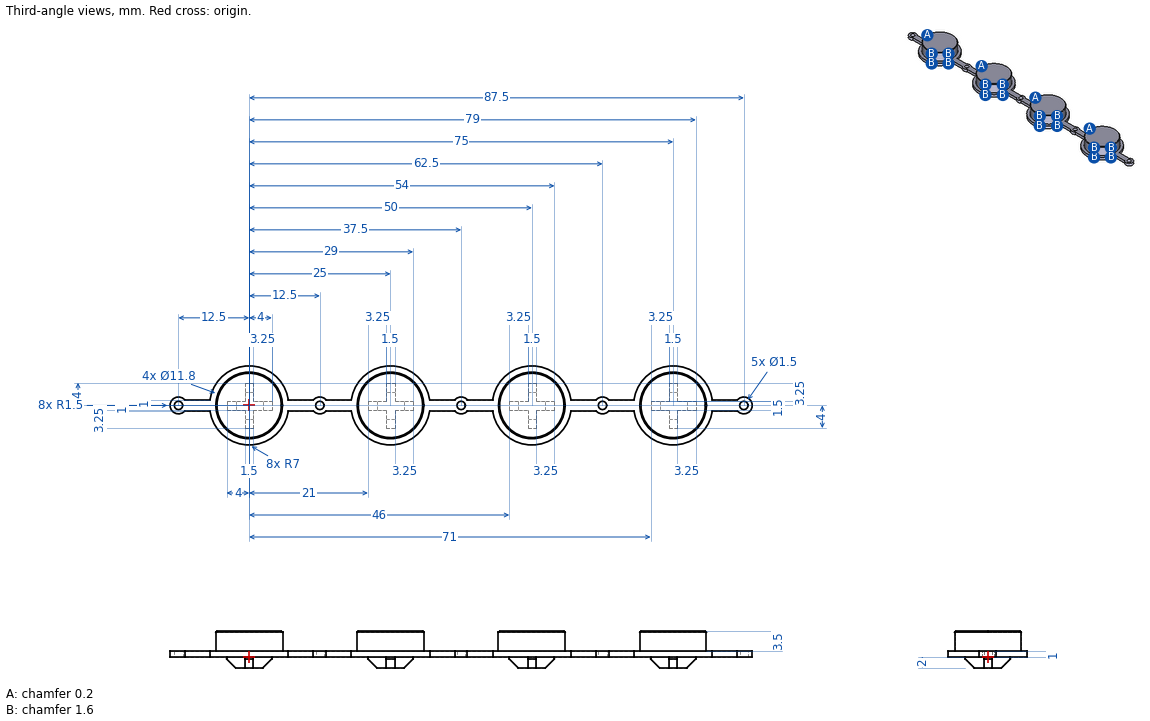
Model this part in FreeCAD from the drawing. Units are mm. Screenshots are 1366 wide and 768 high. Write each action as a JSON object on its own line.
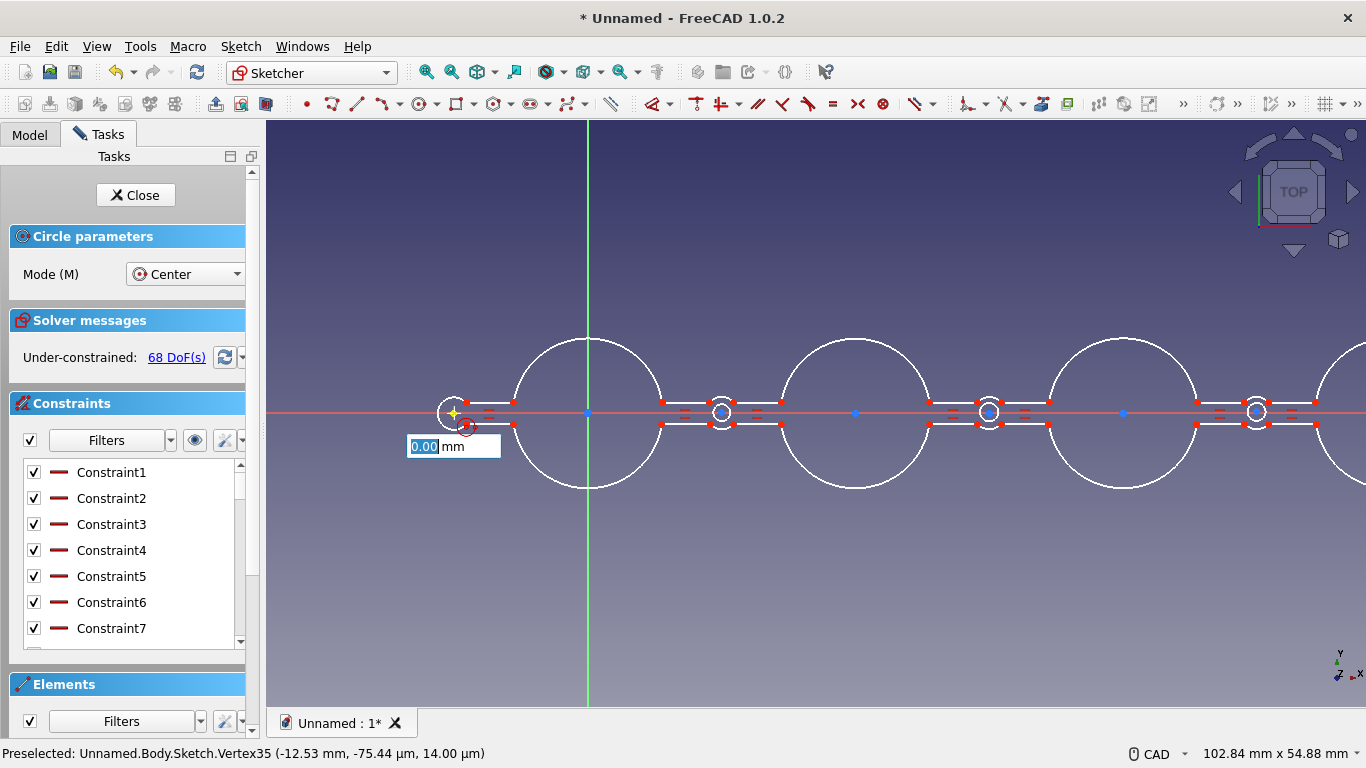
{"action": "scroll", "coordinate": [452, 420], "scroll_direction": "up", "scroll_amount": 4}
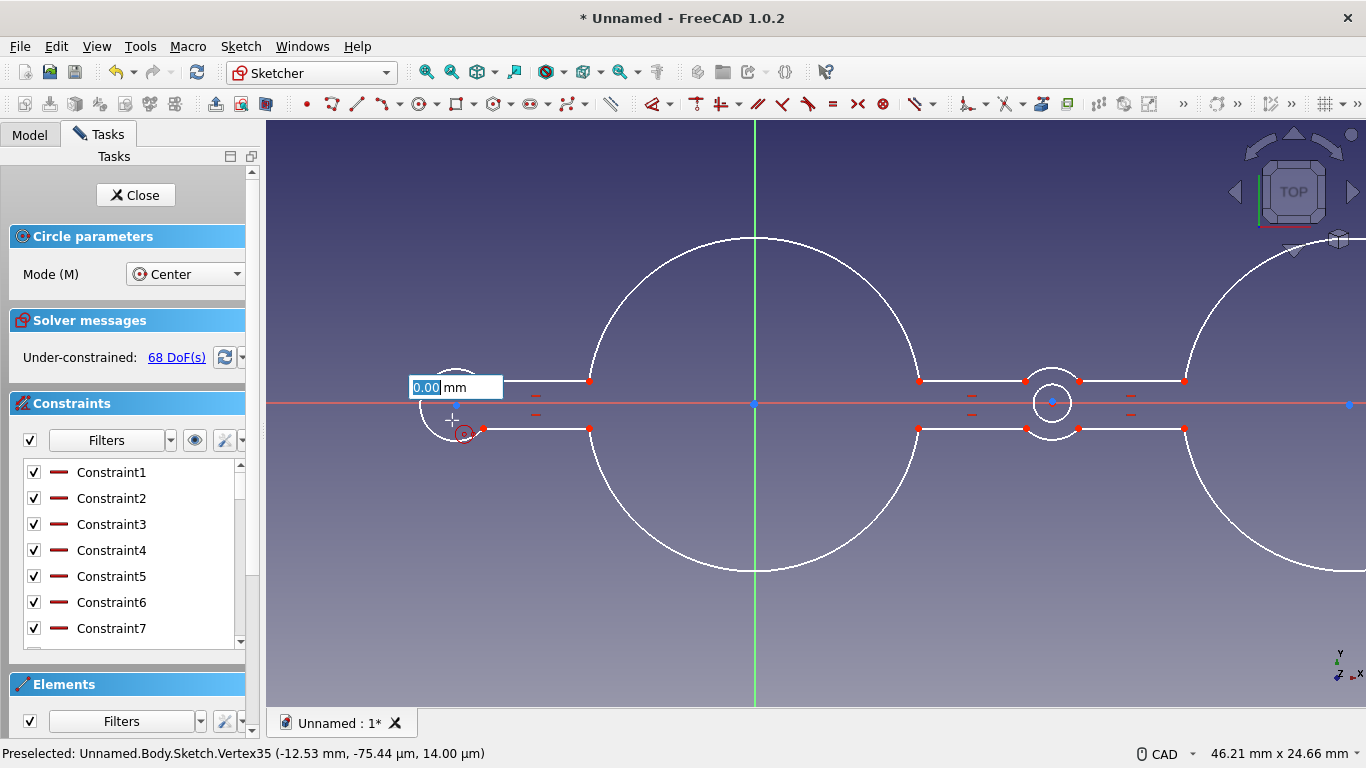
{"action": "left_click", "coordinate": [451, 420]}
{"action": "key", "text": "Escape"}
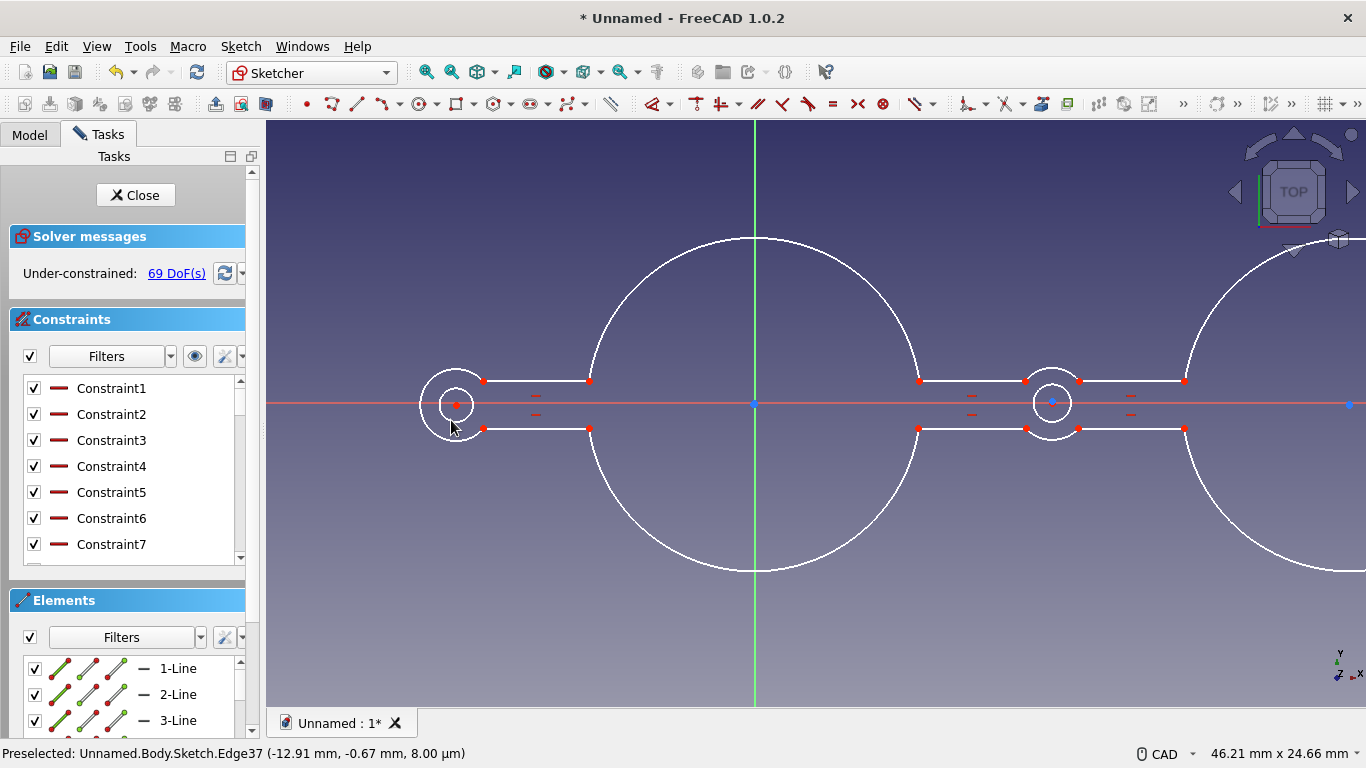
{"action": "scroll", "coordinate": [453, 417], "scroll_direction": "down", "scroll_amount": 7}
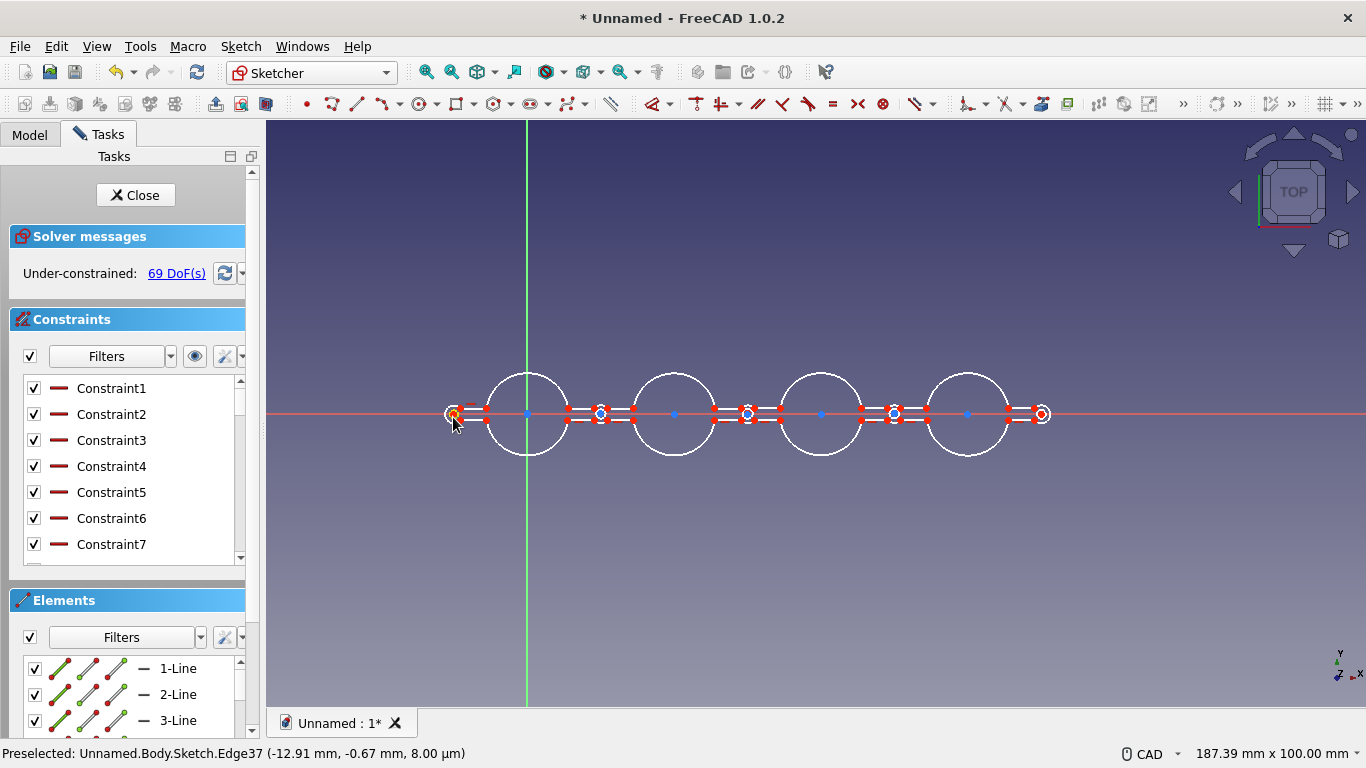
{"action": "left_click", "coordinate": [946, 449]}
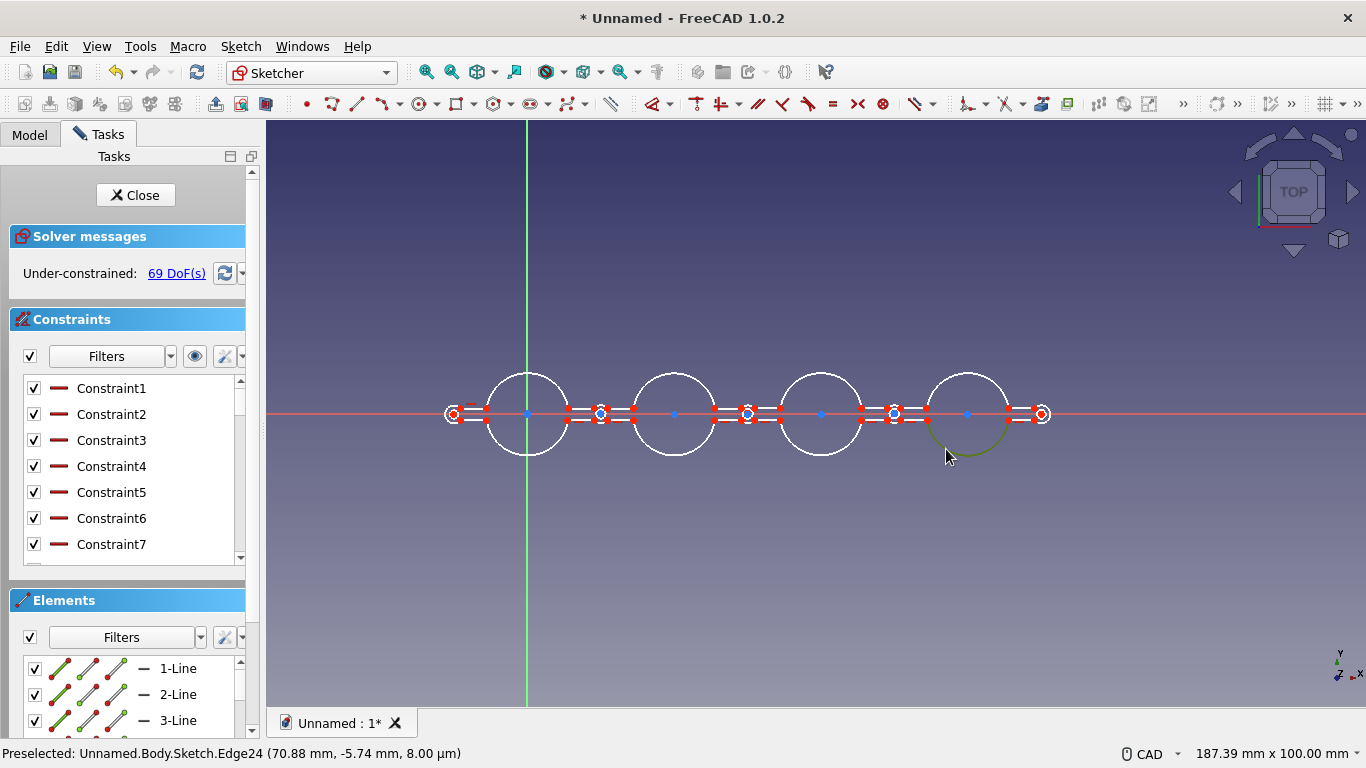
{"action": "left_click", "coordinate": [990, 380]}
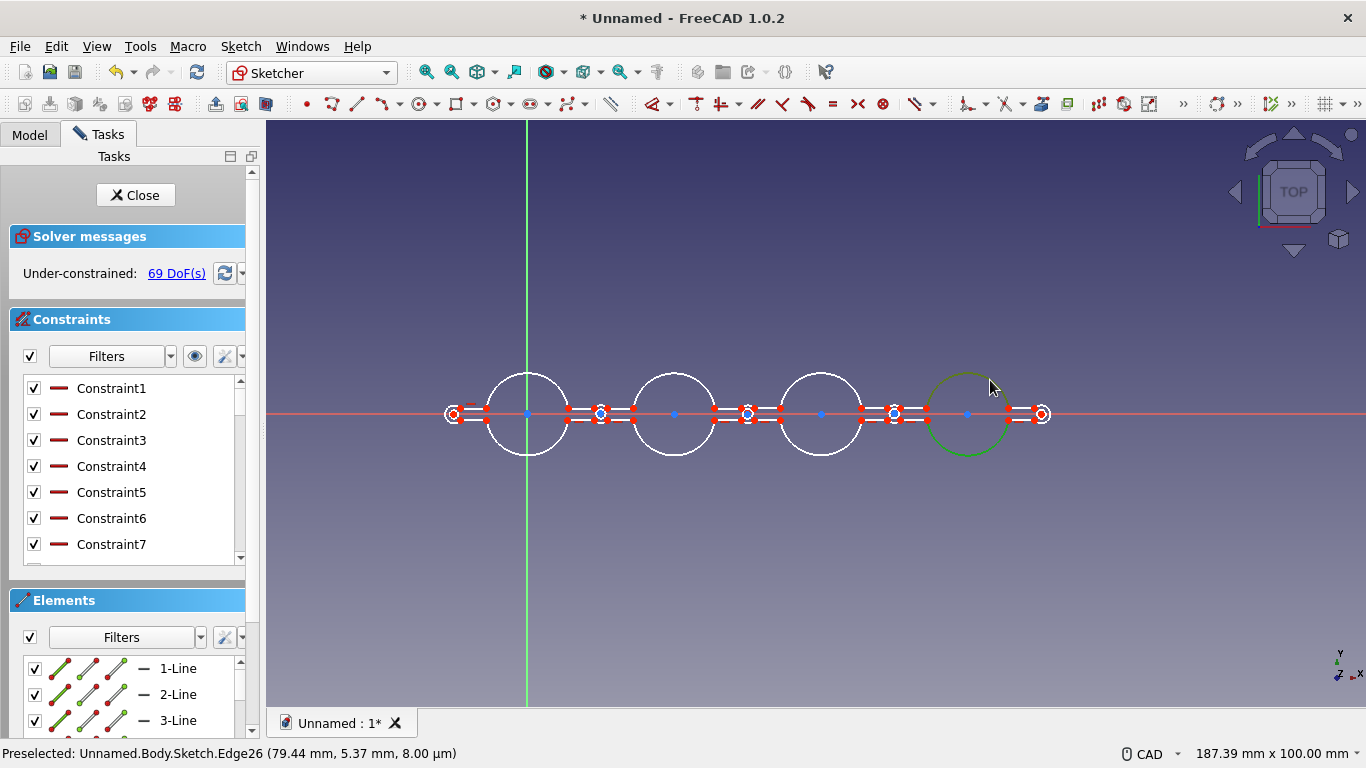
{"action": "left_click", "coordinate": [696, 104]}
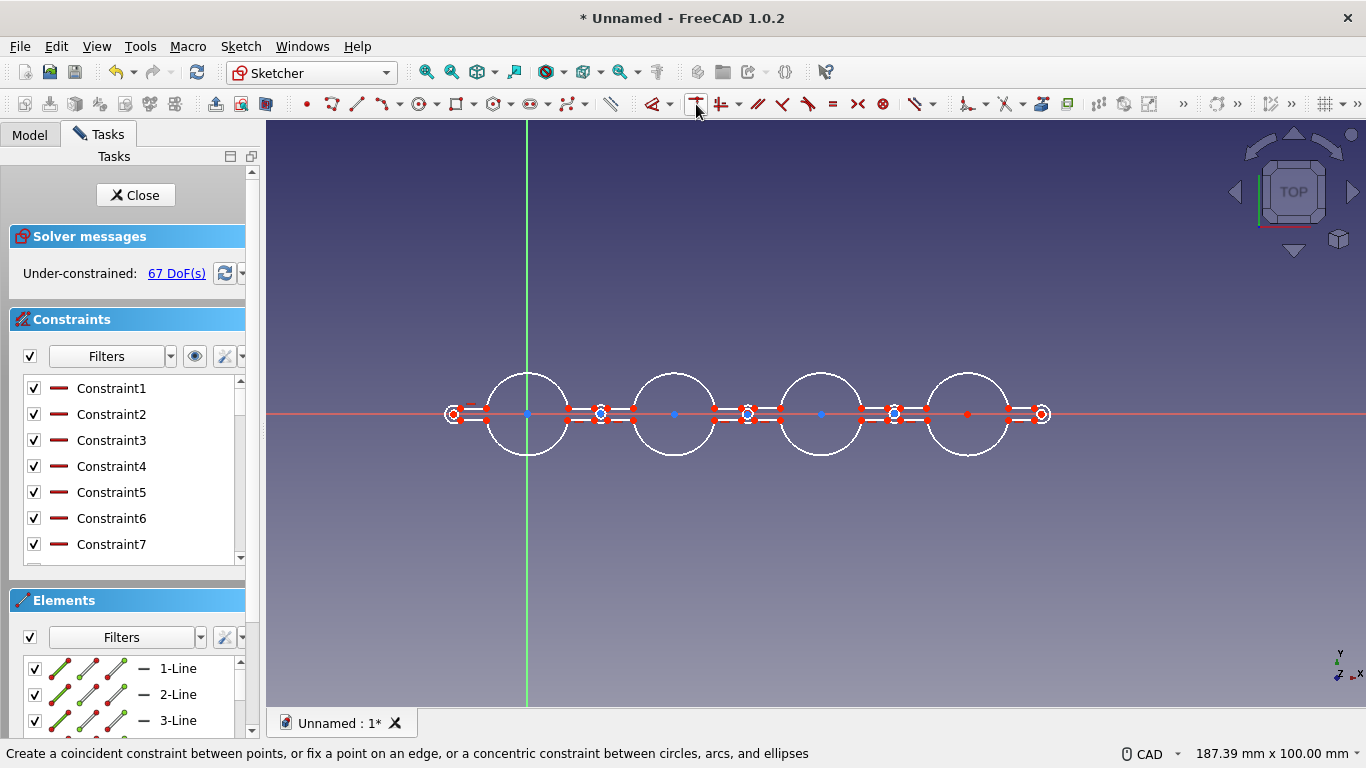
{"action": "scroll", "coordinate": [889, 413], "scroll_direction": "up", "scroll_amount": 6}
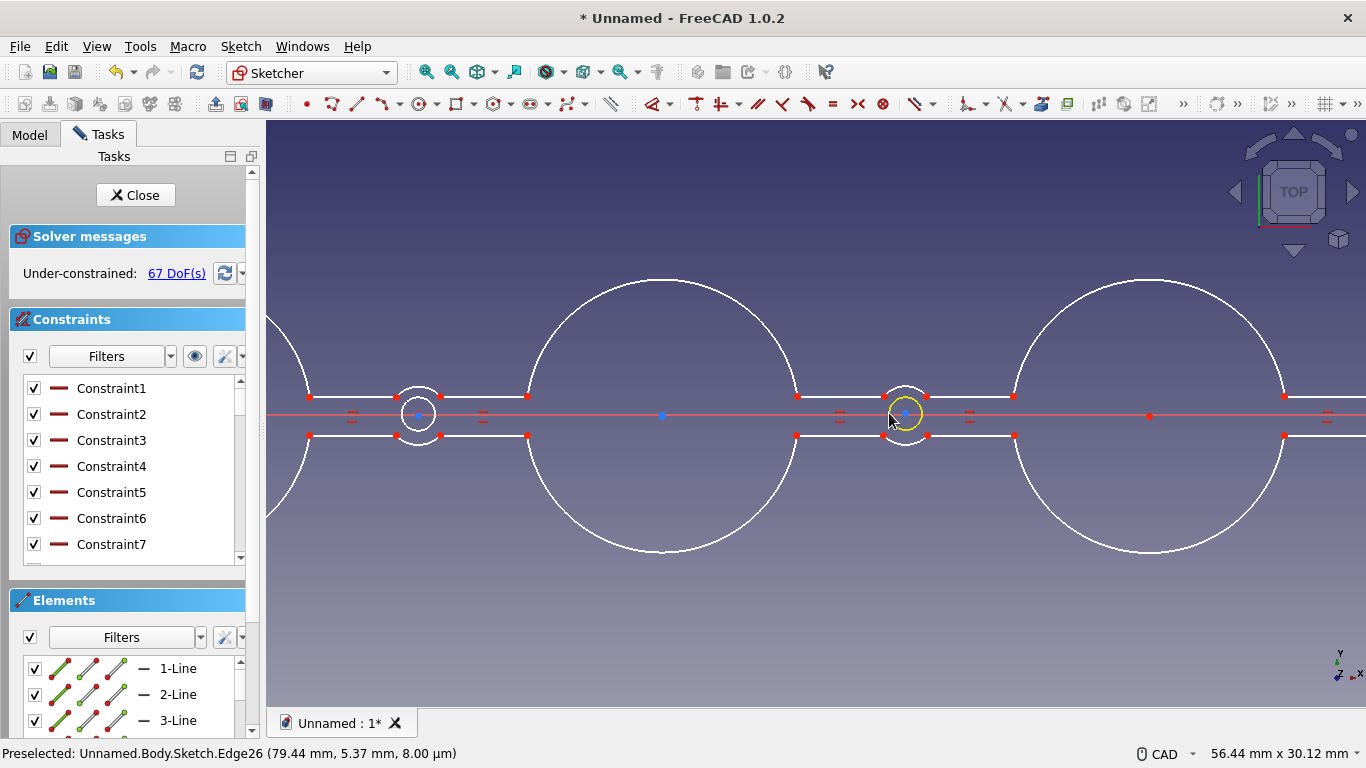
{"action": "left_click", "coordinate": [889, 413]}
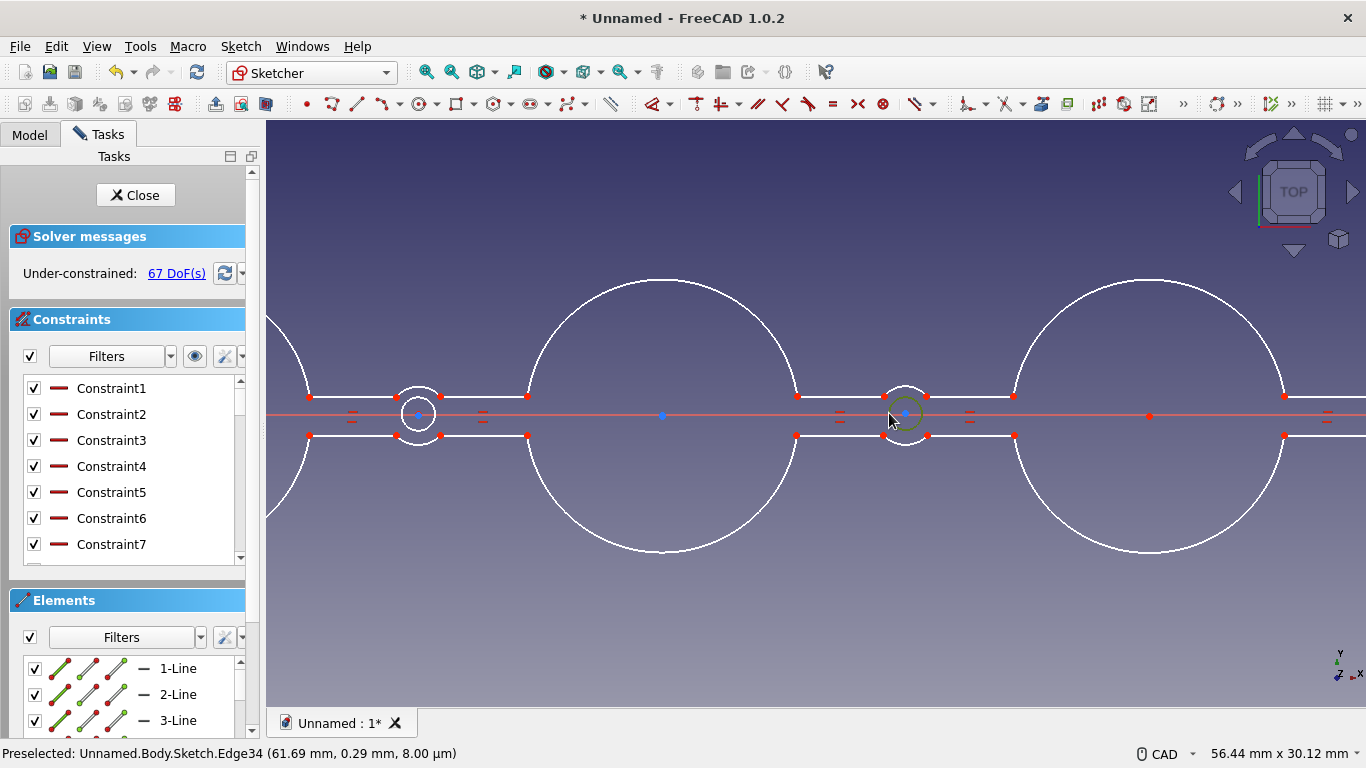
{"action": "scroll", "coordinate": [915, 388], "scroll_direction": "up", "scroll_amount": 2}